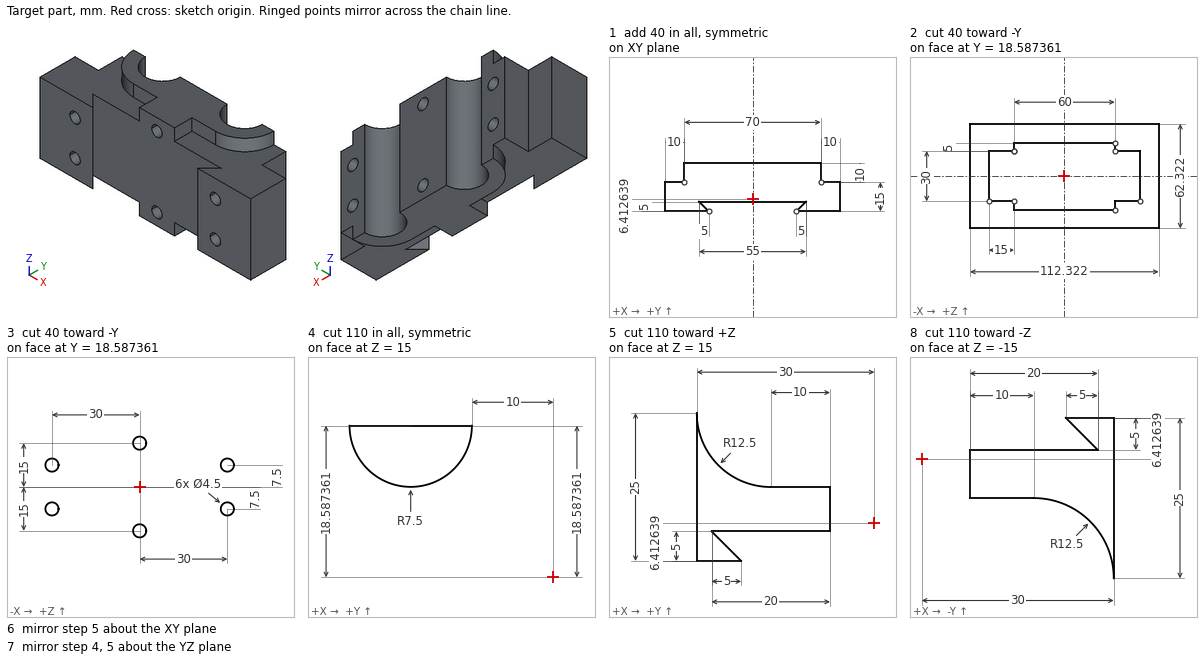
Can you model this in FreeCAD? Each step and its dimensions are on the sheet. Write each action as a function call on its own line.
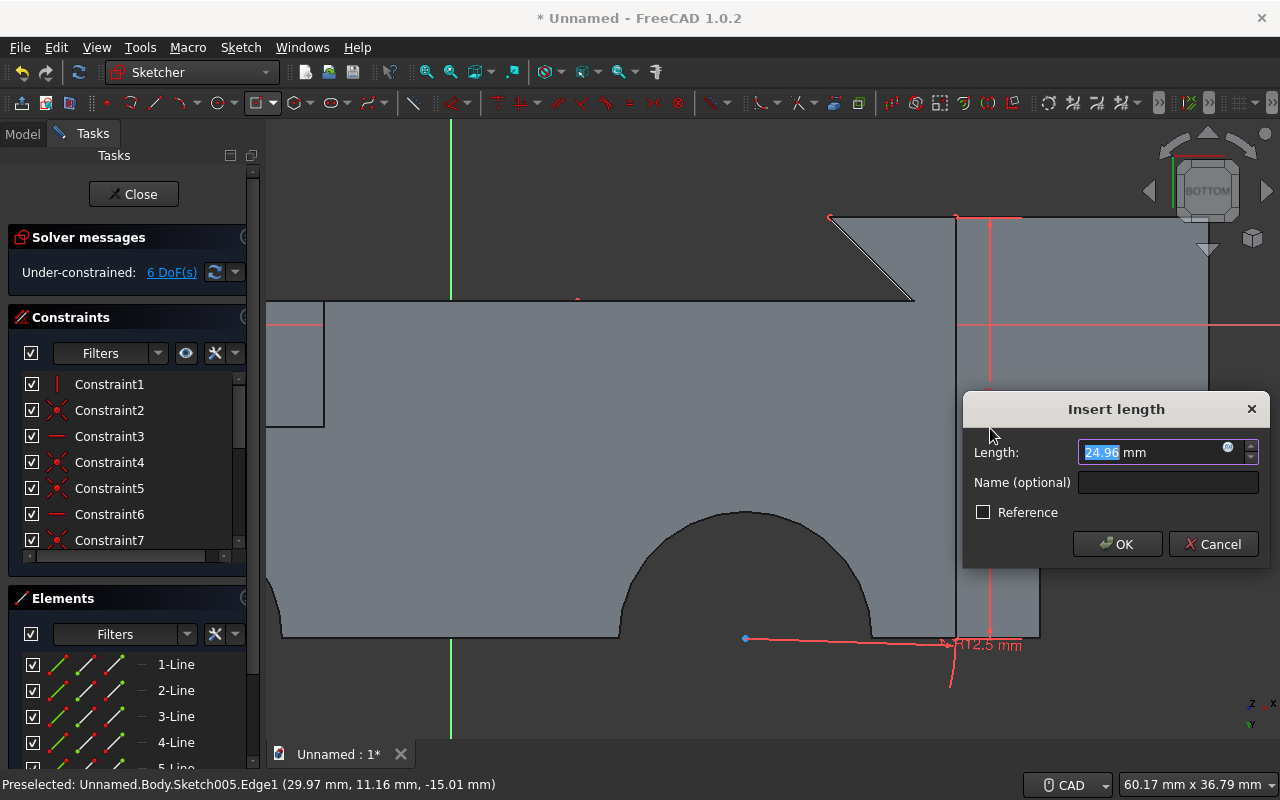
text(25)
key(Return)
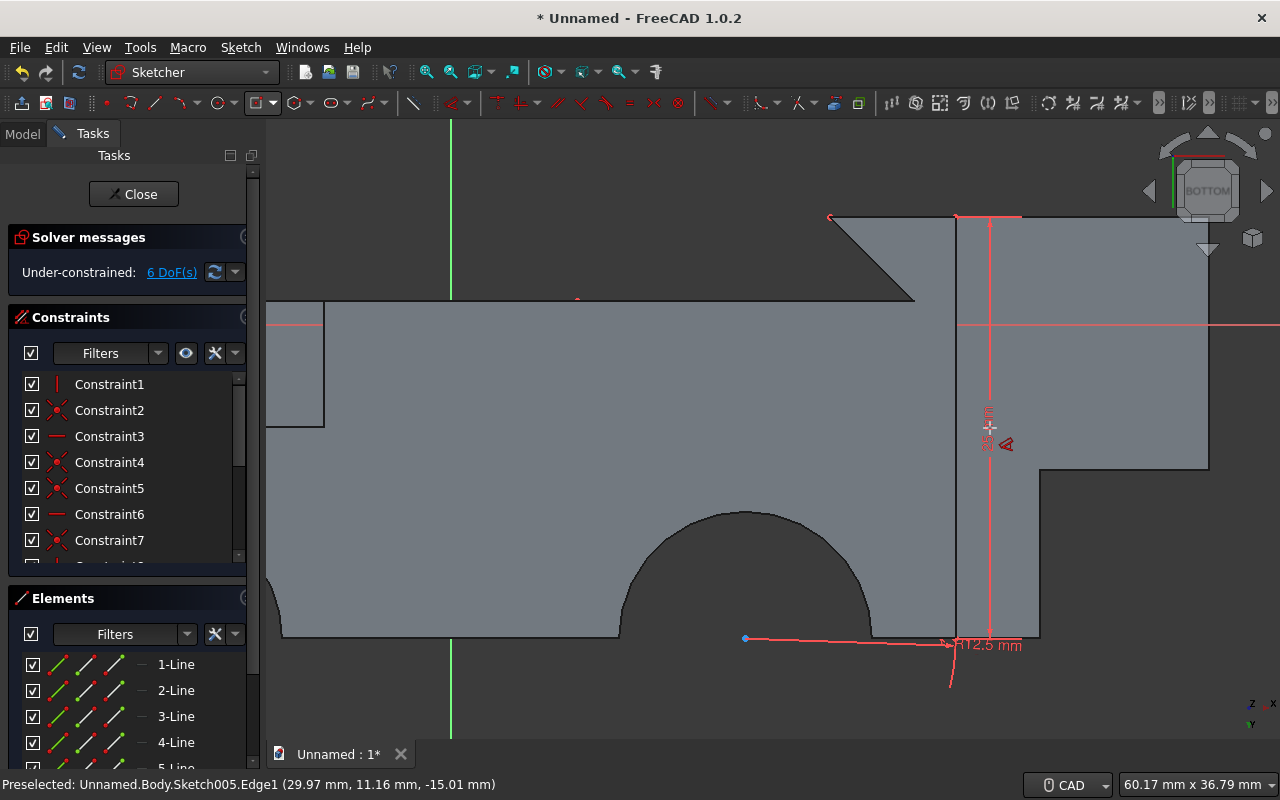
click(813, 302)
click(745, 268)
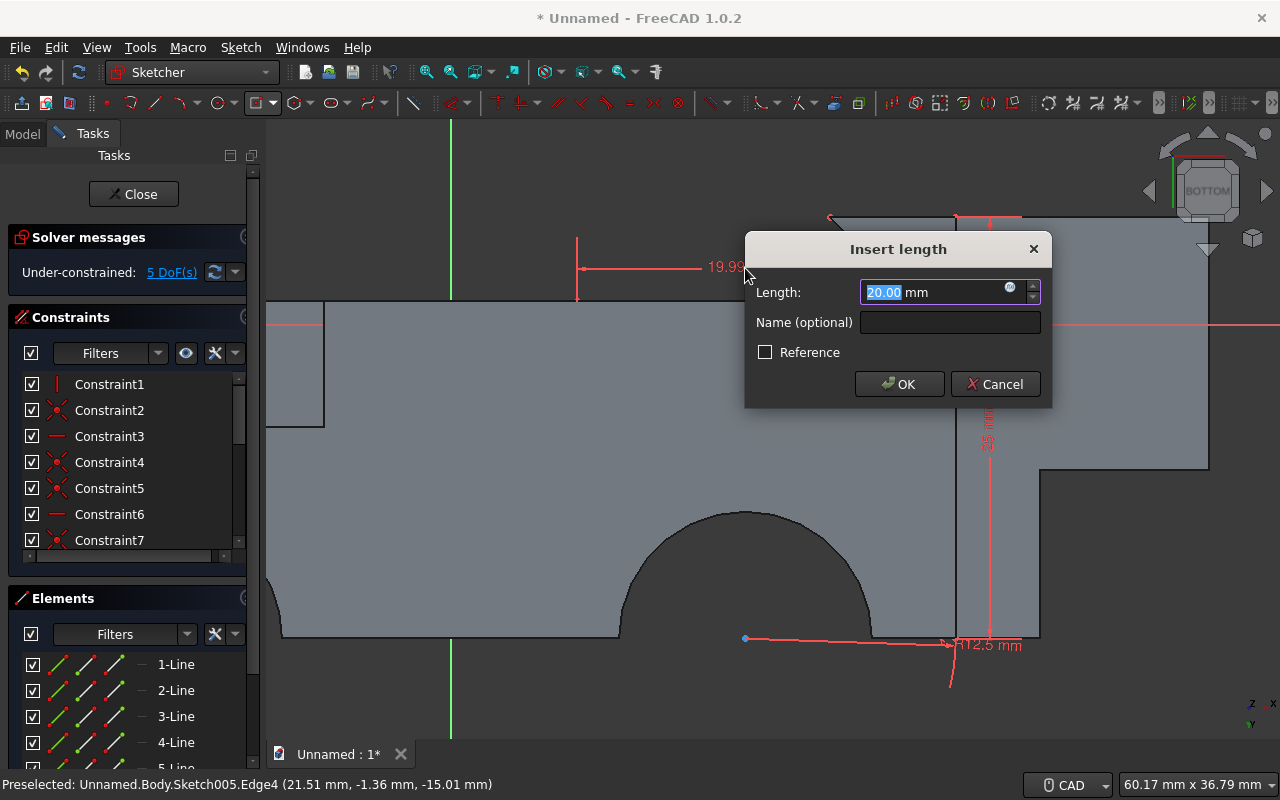
text(20)
key(Return)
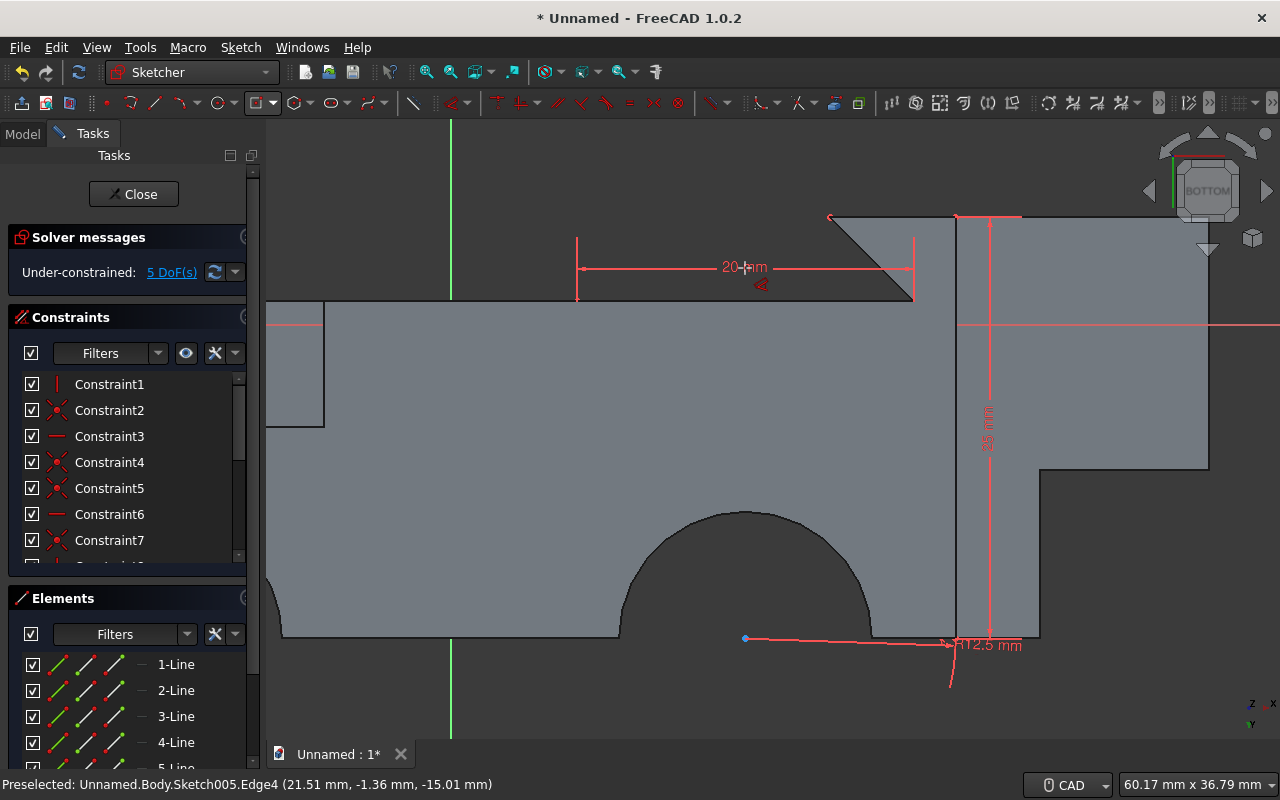
click(627, 428)
click(661, 462)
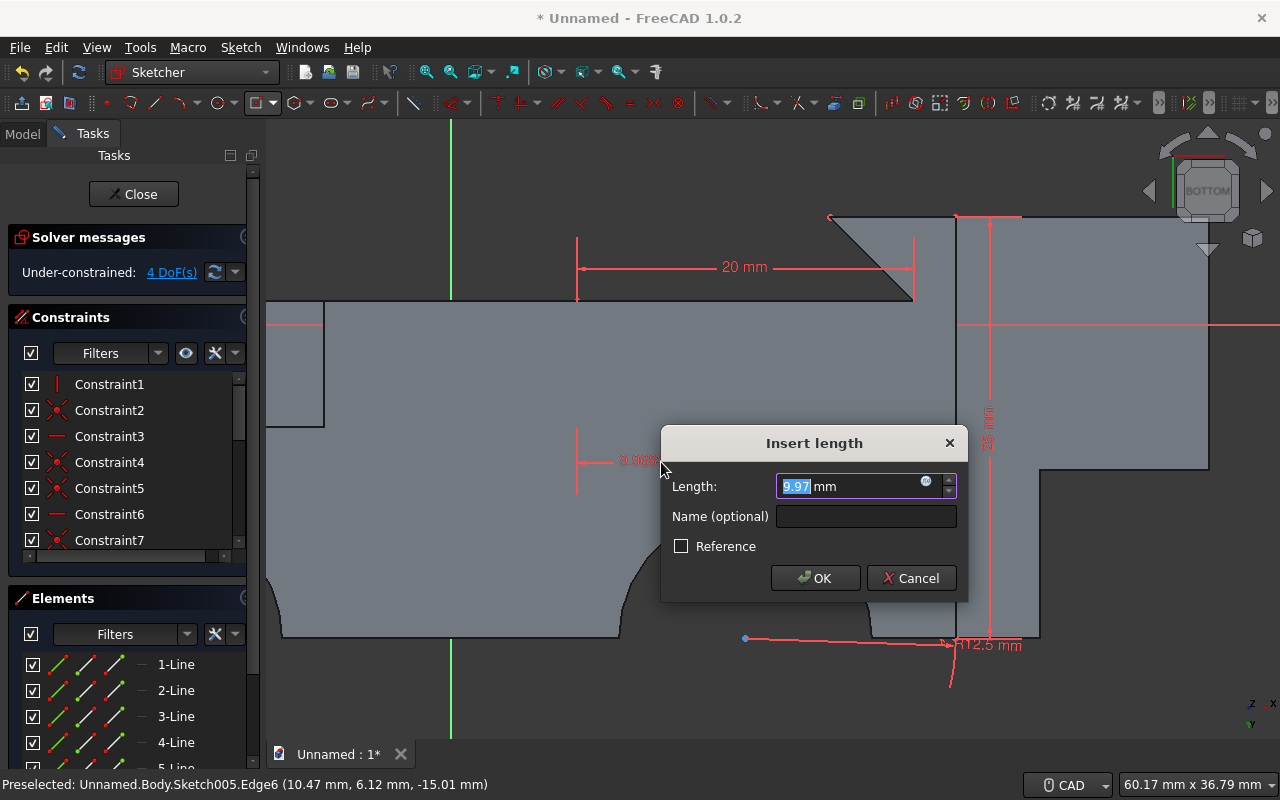
text(10)
key(Return)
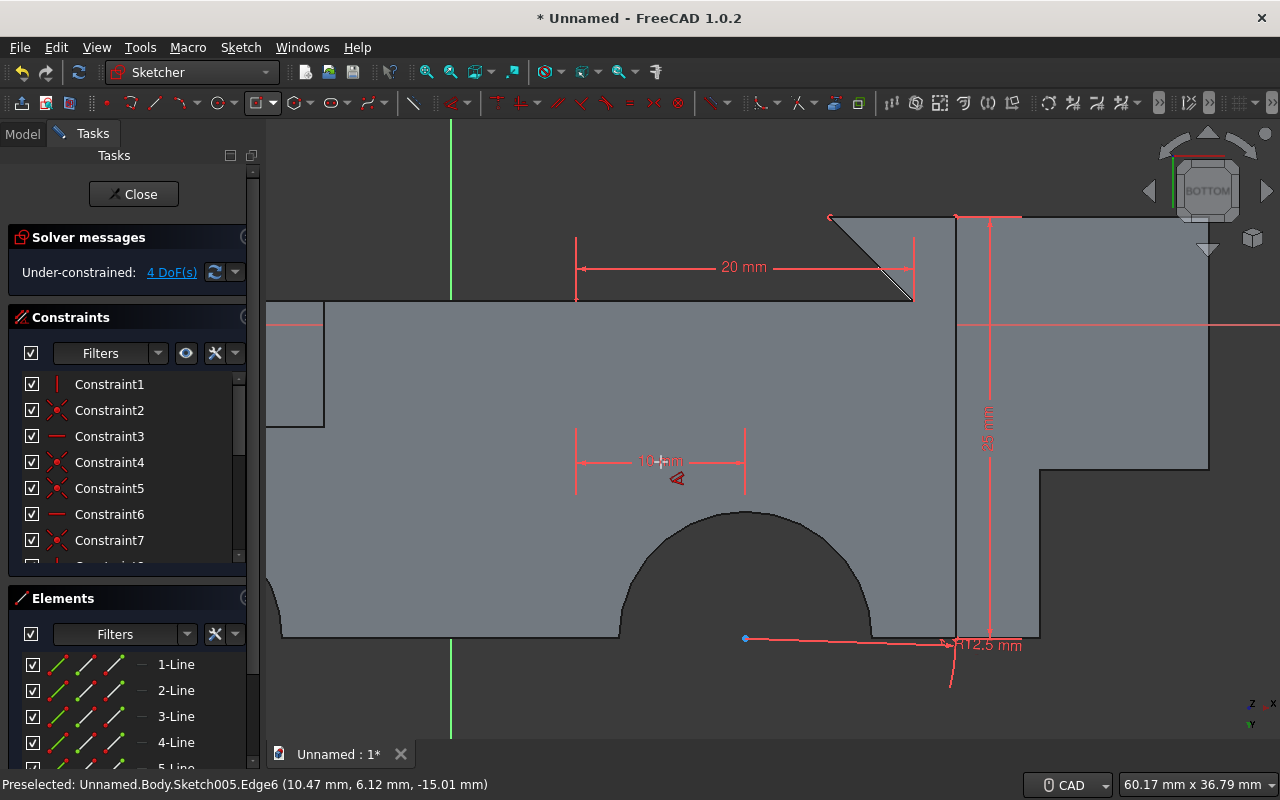
click(855, 243)
click(872, 183)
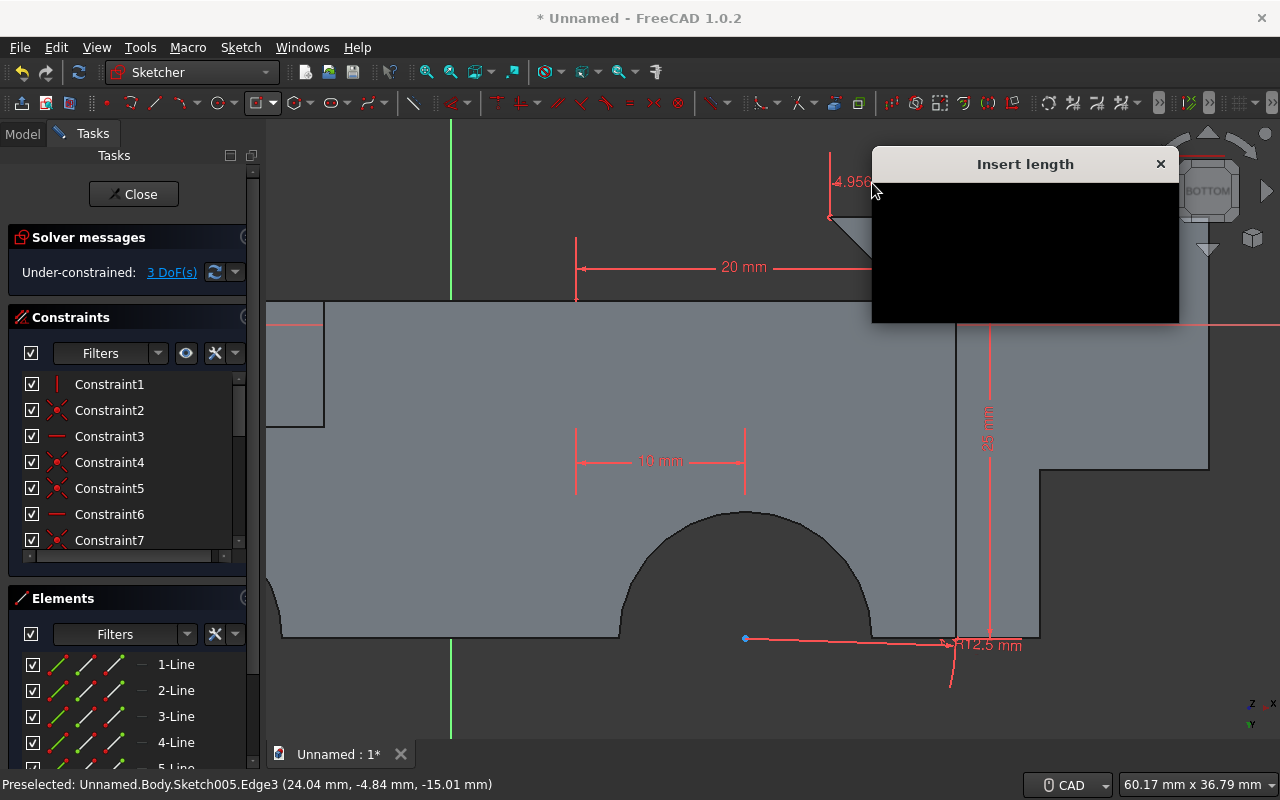
text(5)
key(Return)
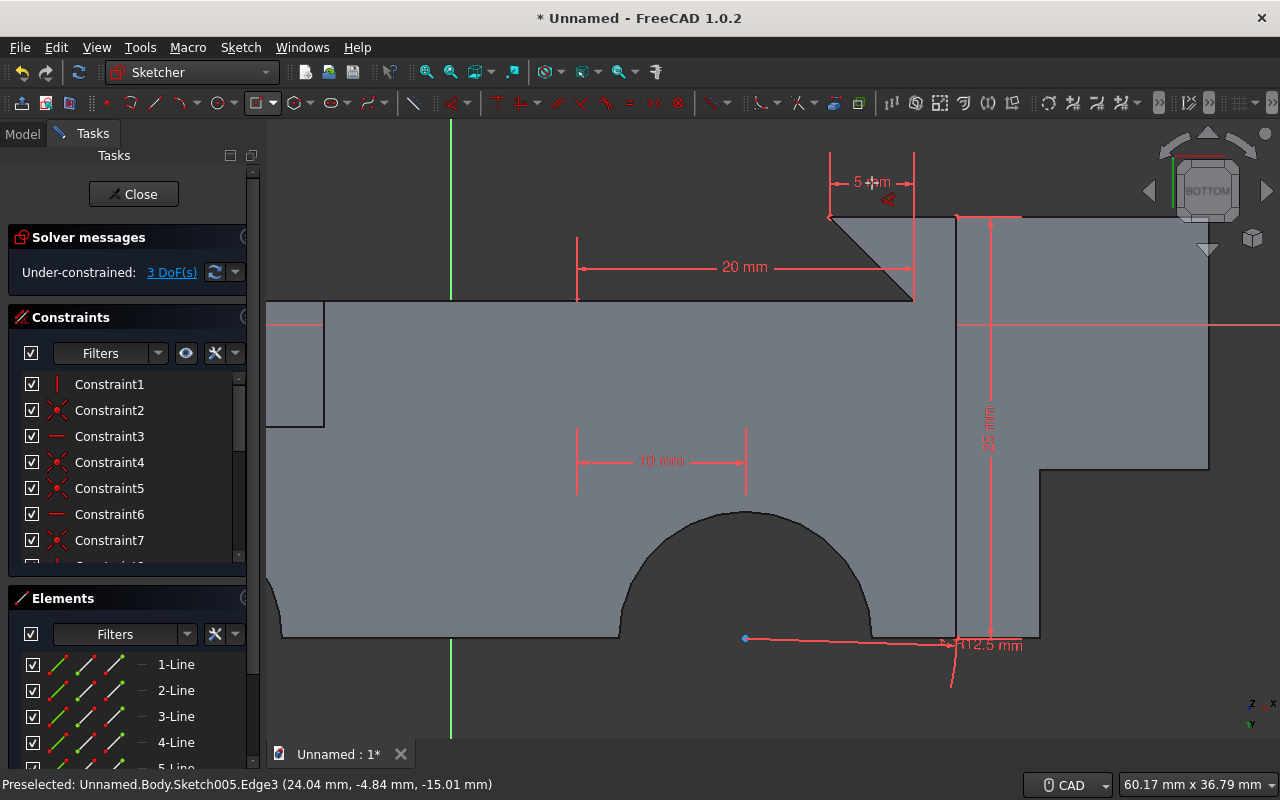
click(855, 243)
click(796, 240)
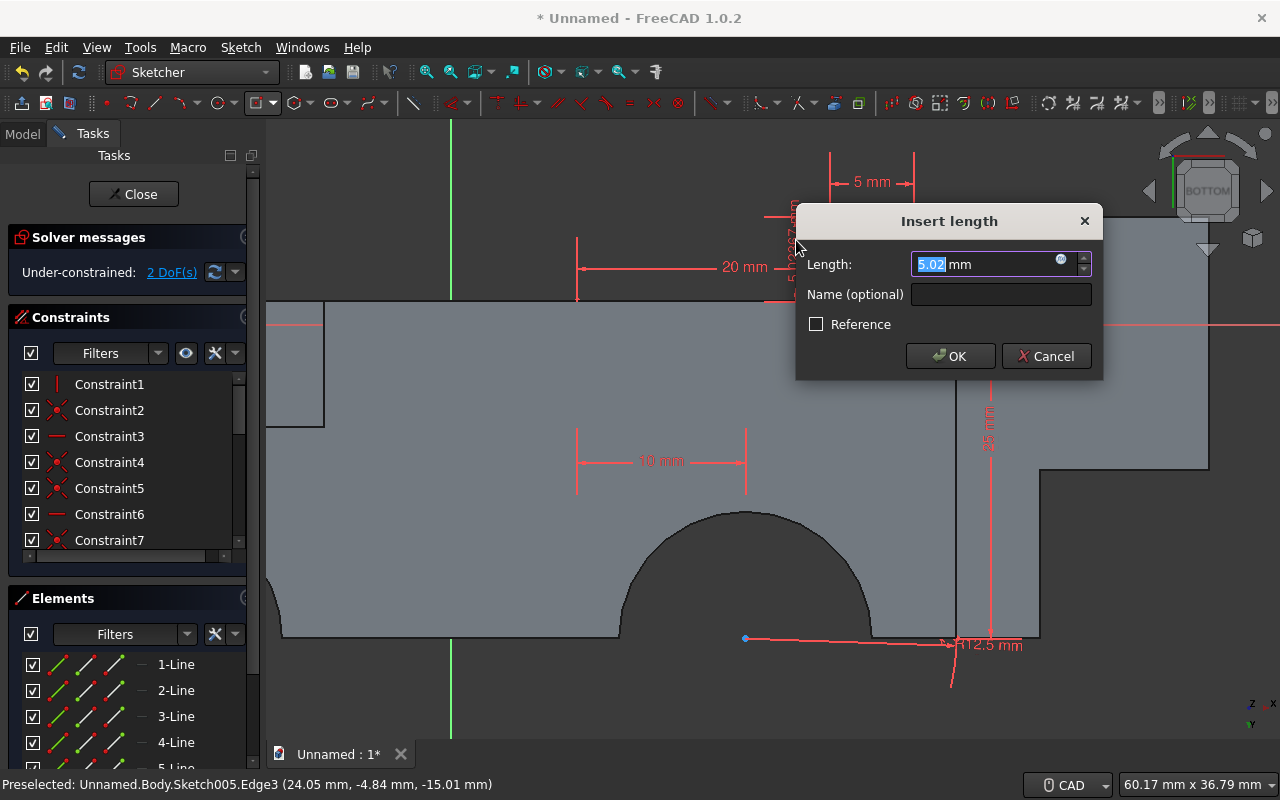
text(5)
key(Return)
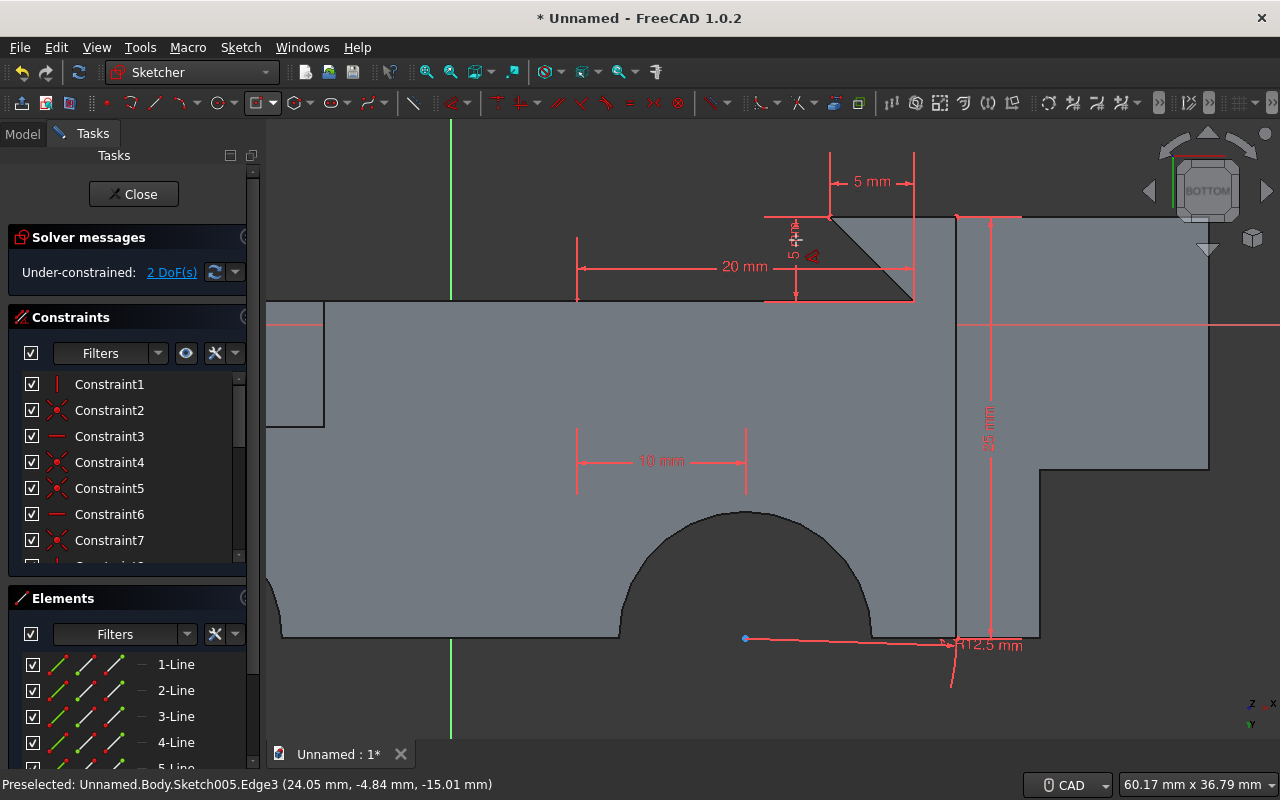
click(956, 639)
click(703, 673)